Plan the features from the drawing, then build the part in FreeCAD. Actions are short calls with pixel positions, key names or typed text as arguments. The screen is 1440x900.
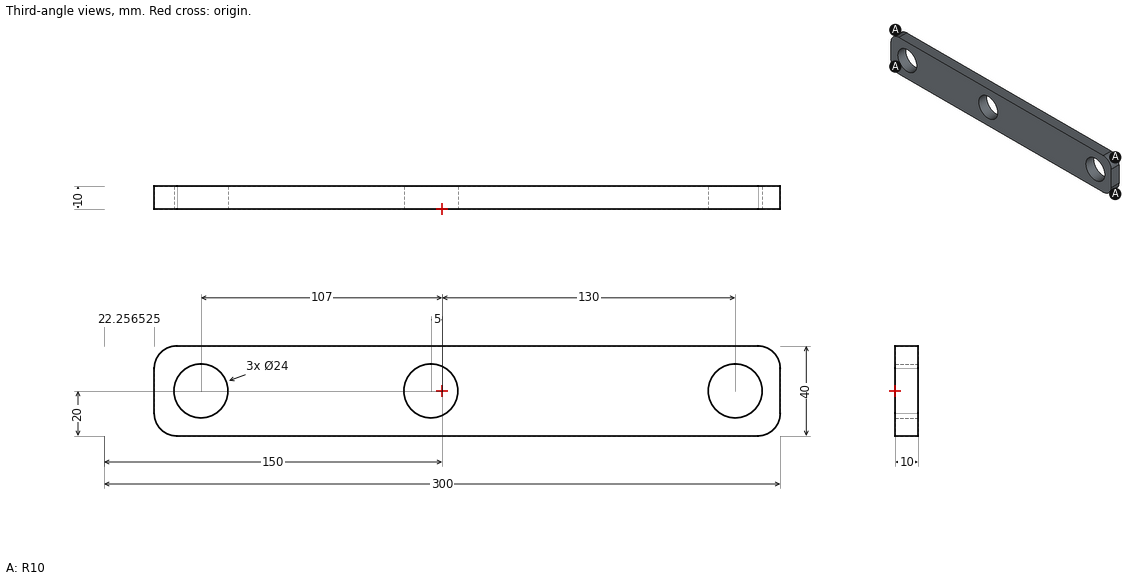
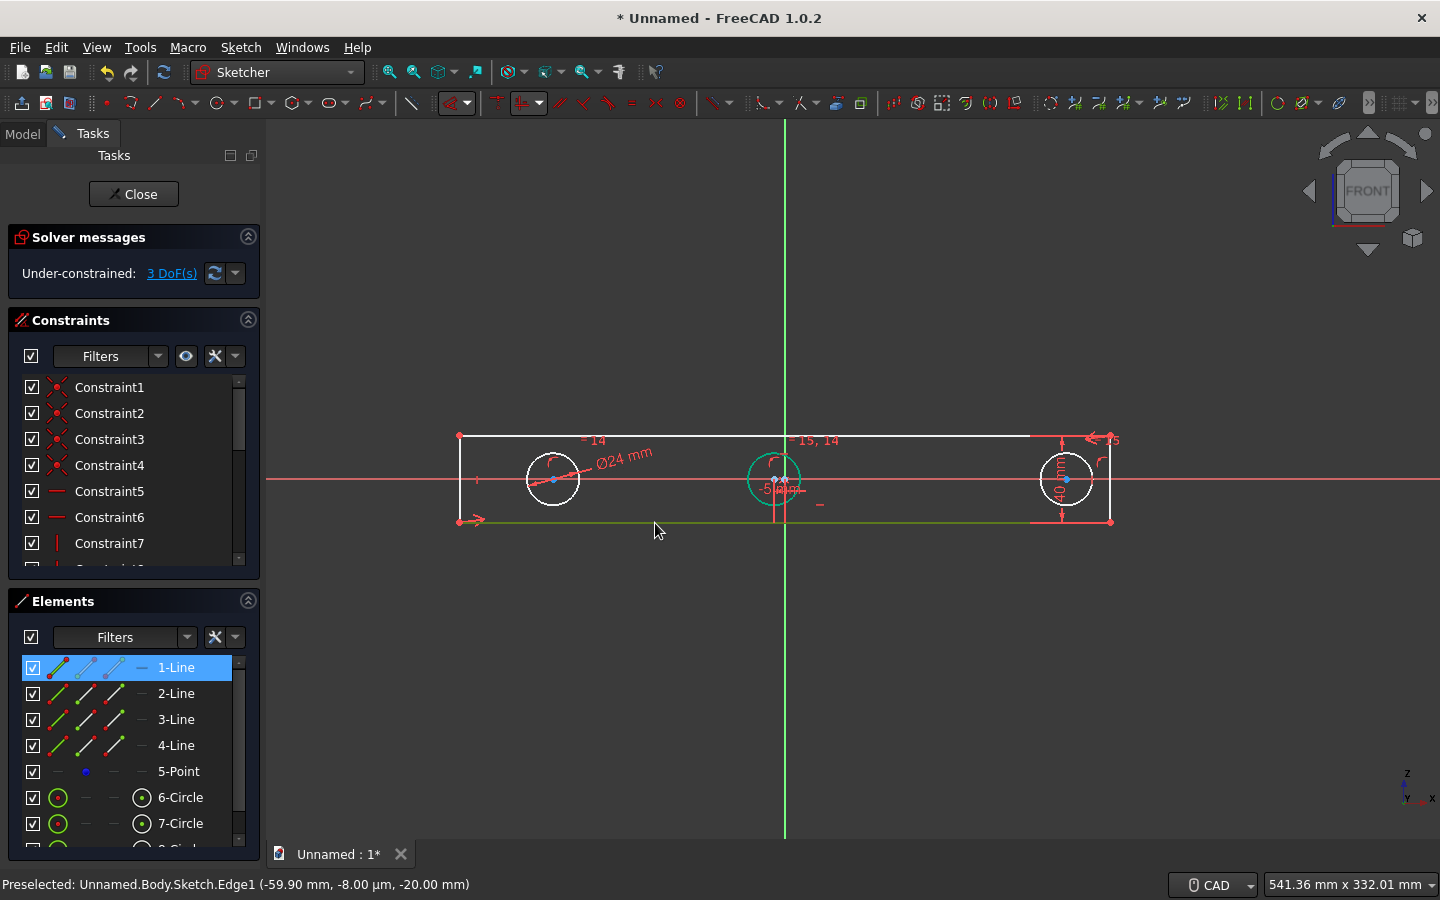
key(l)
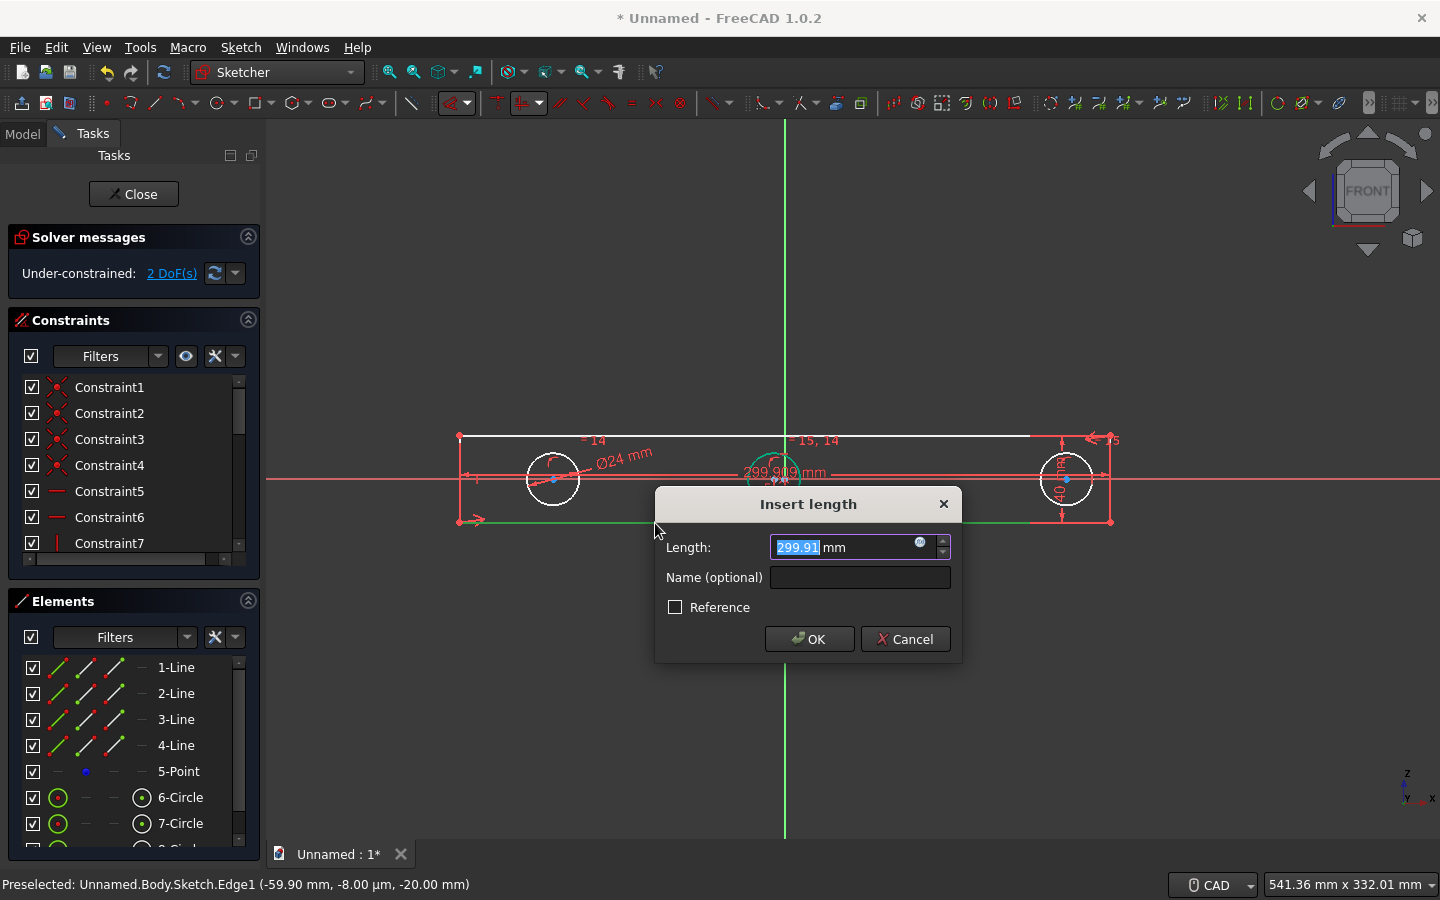
text(300)
key(Return)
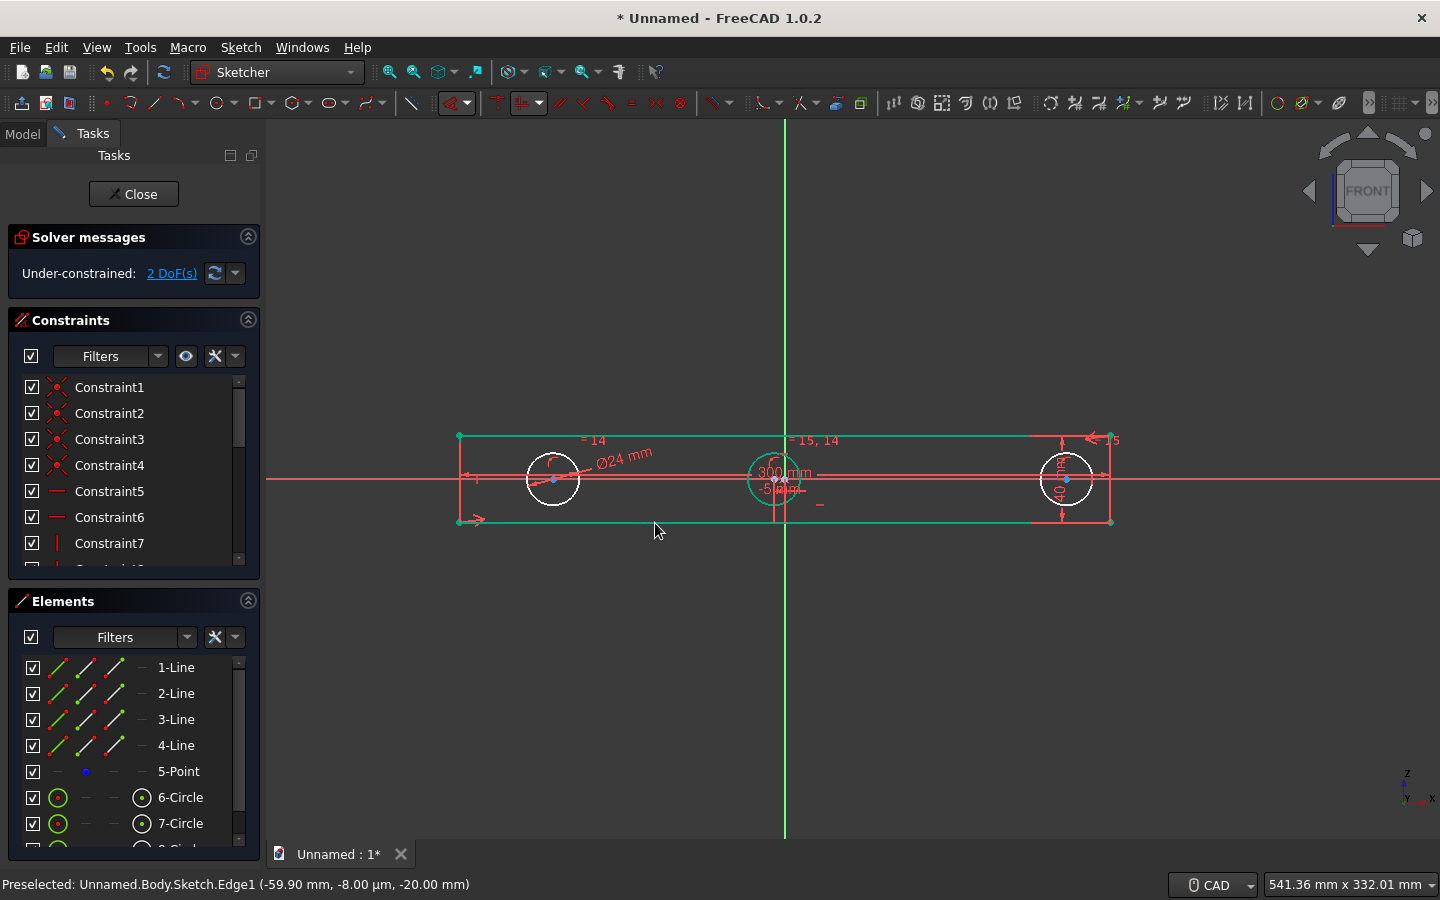
click(553, 479)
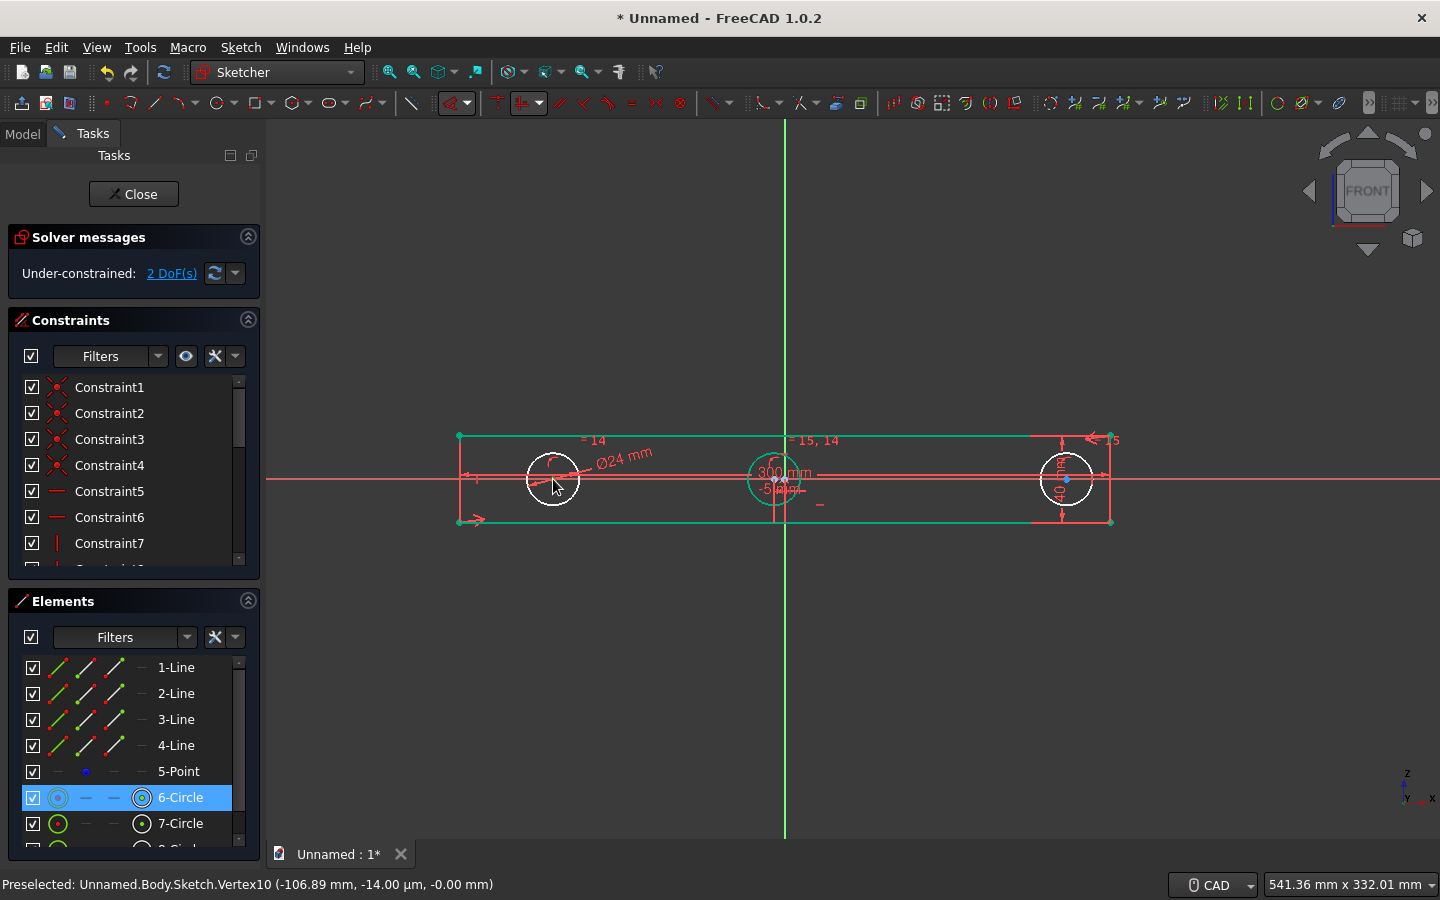
key(l)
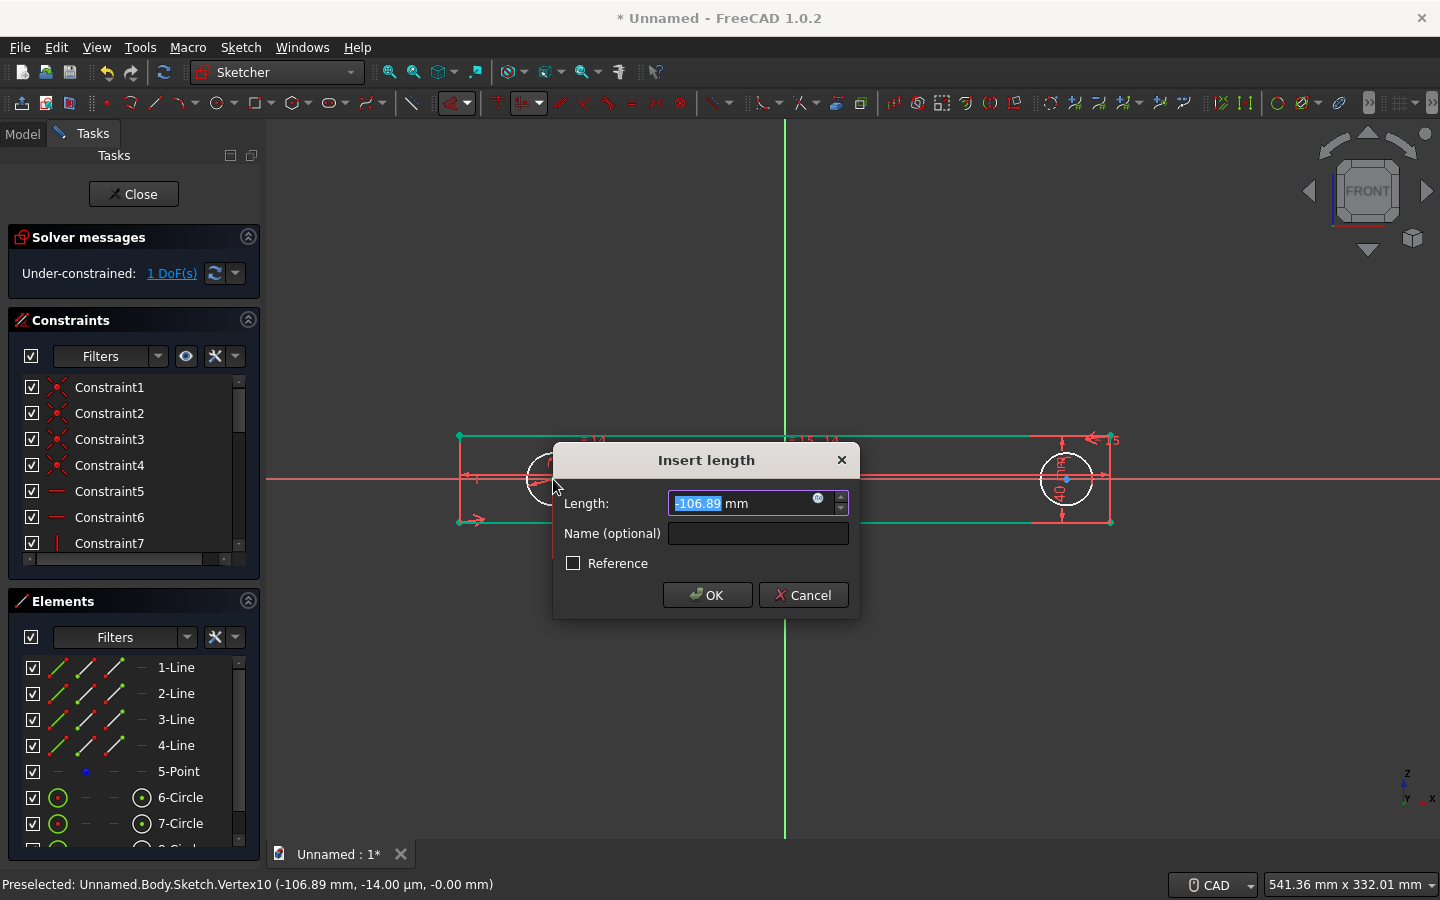
text(-107)
key(Return)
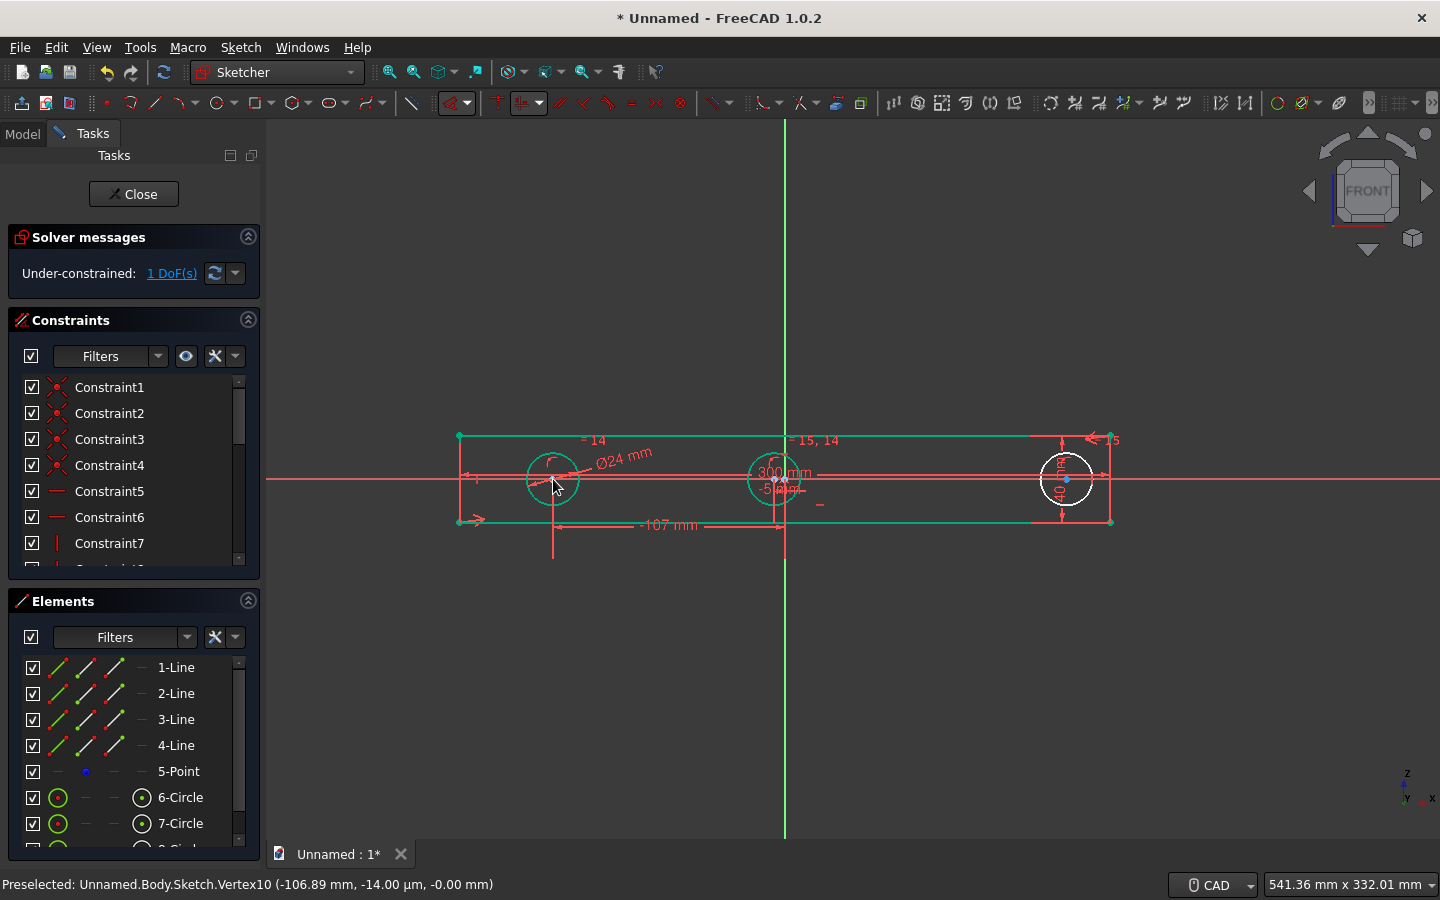
click(1066, 479)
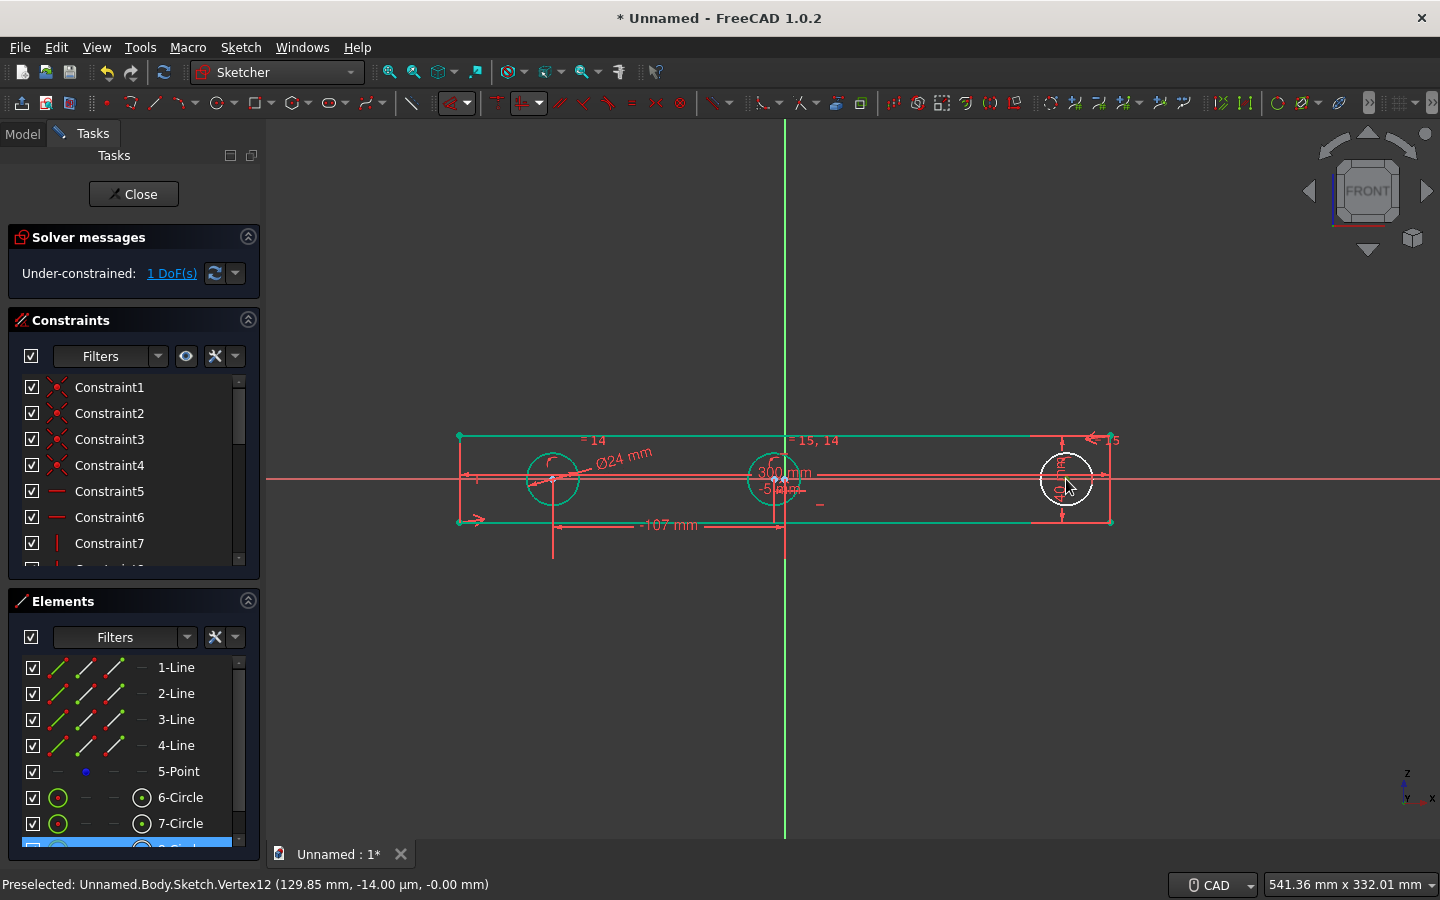
click(470, 104)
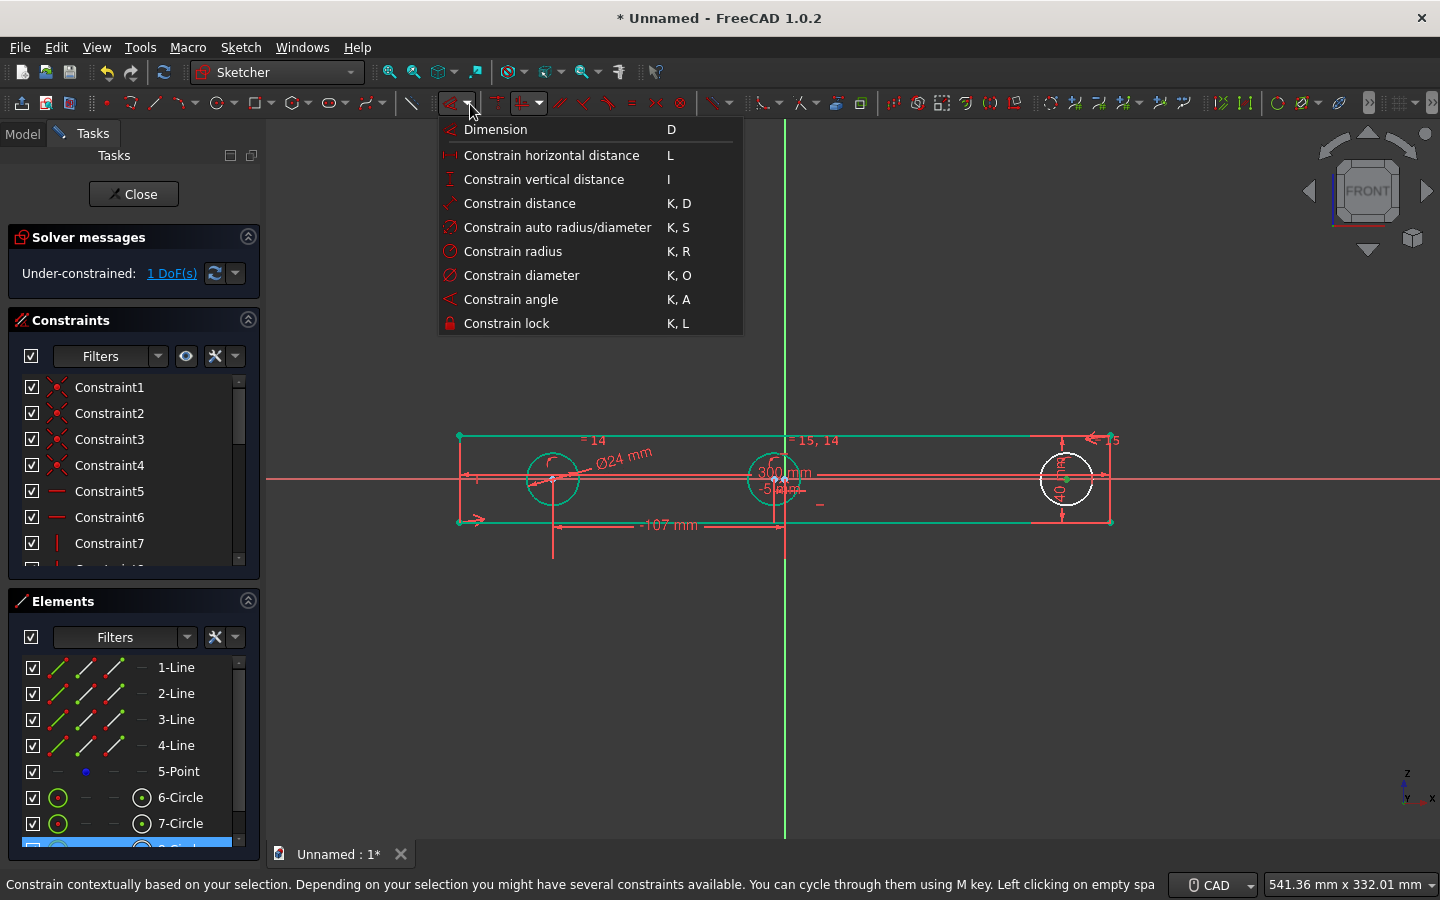
click(591, 155)